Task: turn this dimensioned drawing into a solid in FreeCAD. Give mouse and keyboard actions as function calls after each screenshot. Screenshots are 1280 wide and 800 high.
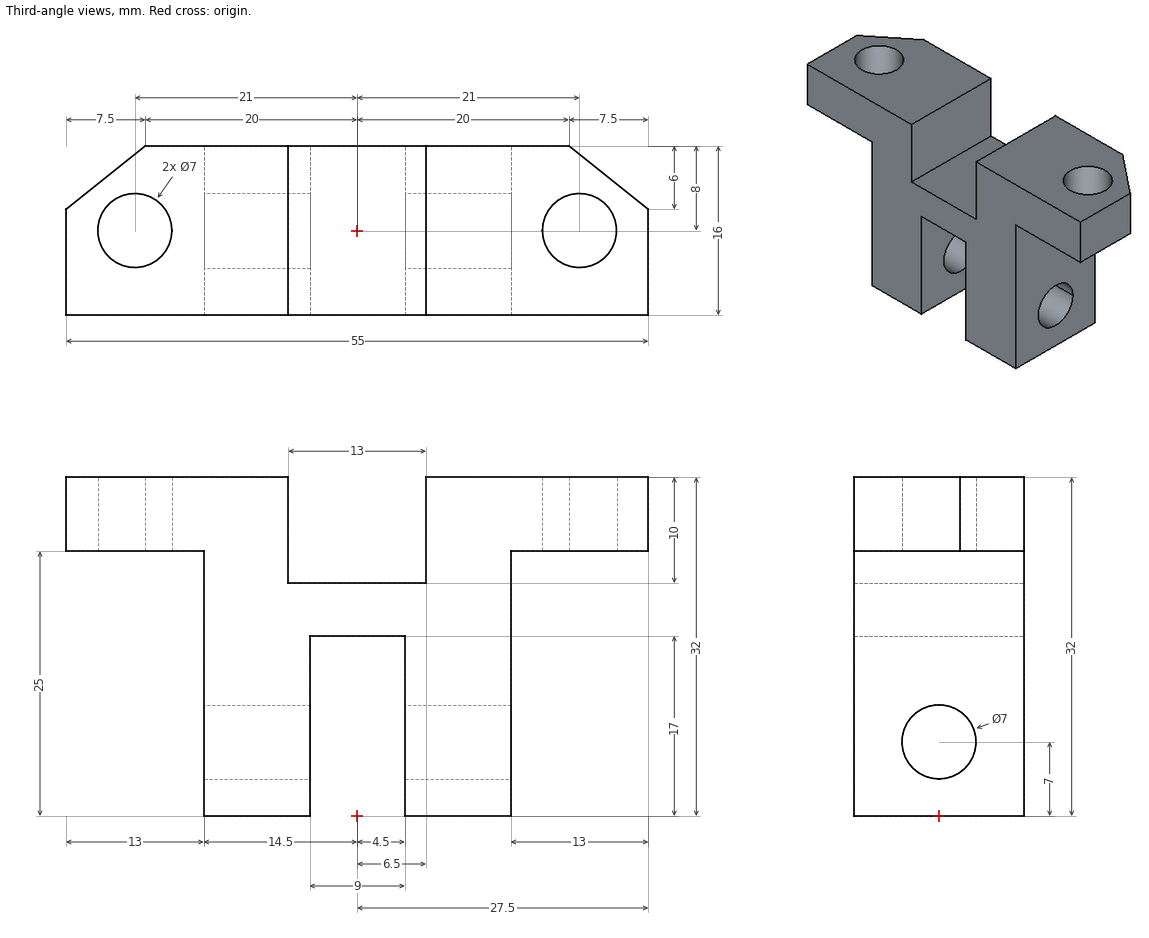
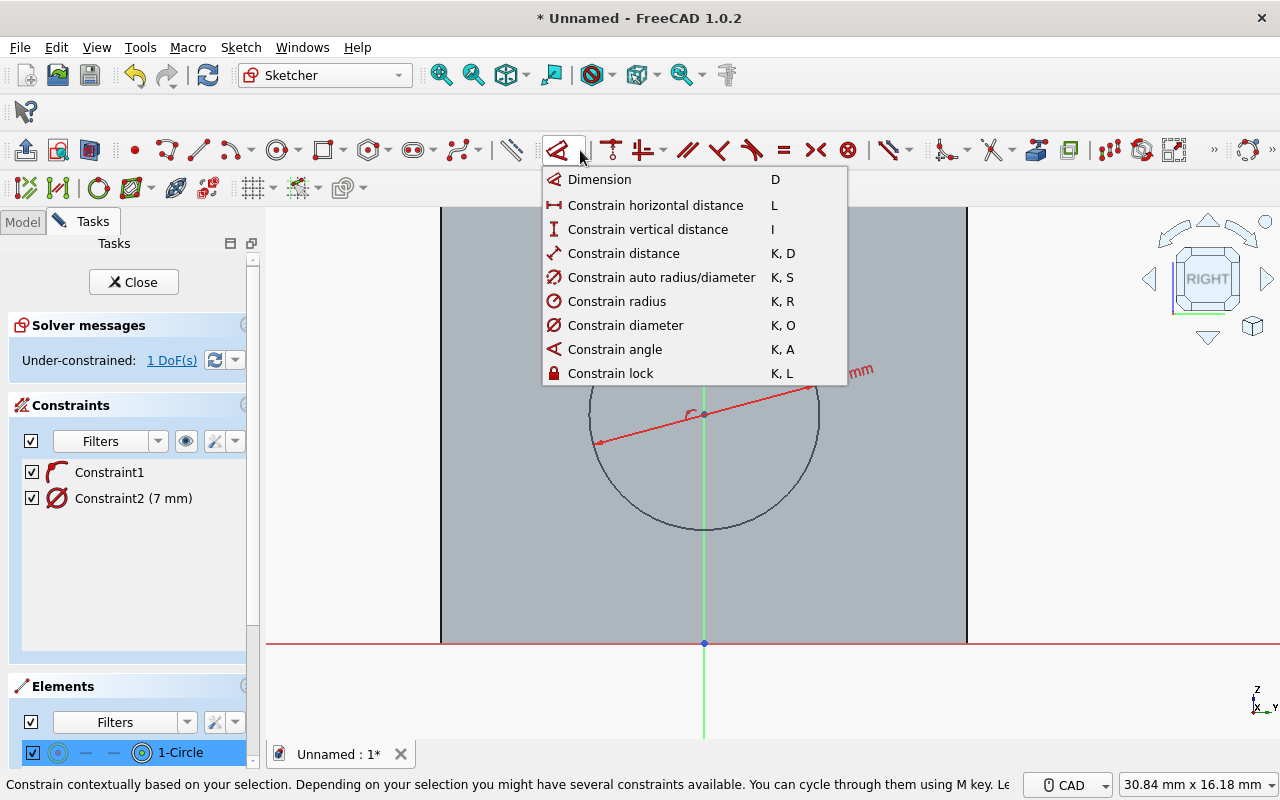
click(695, 229)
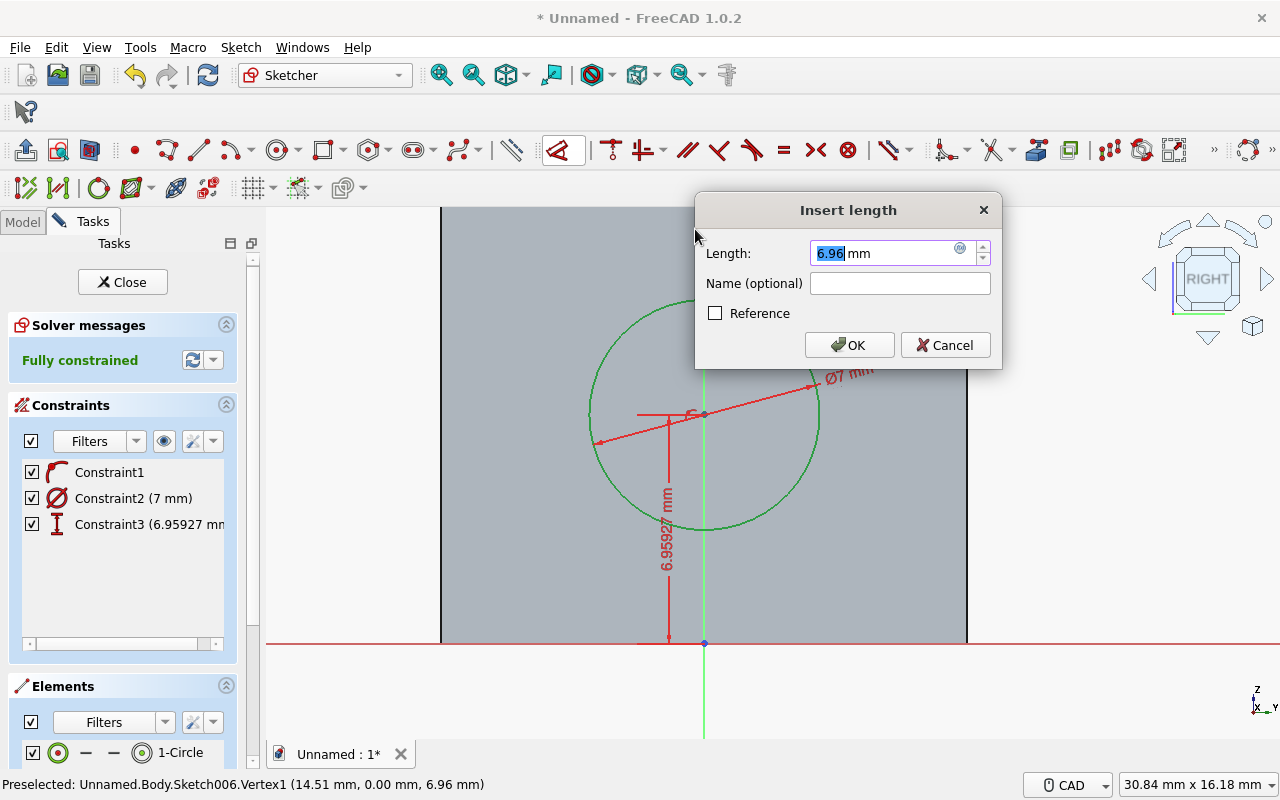
text(7)
key(Return)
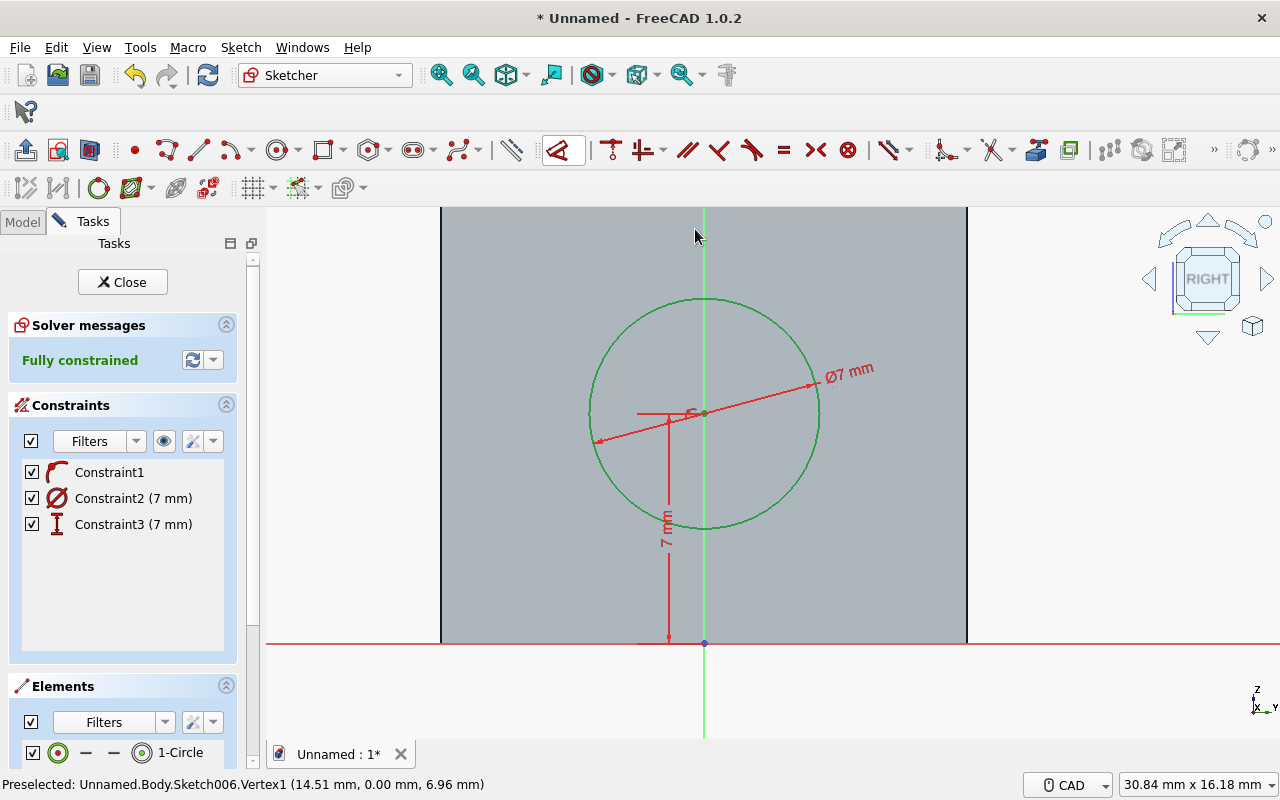
click(123, 282)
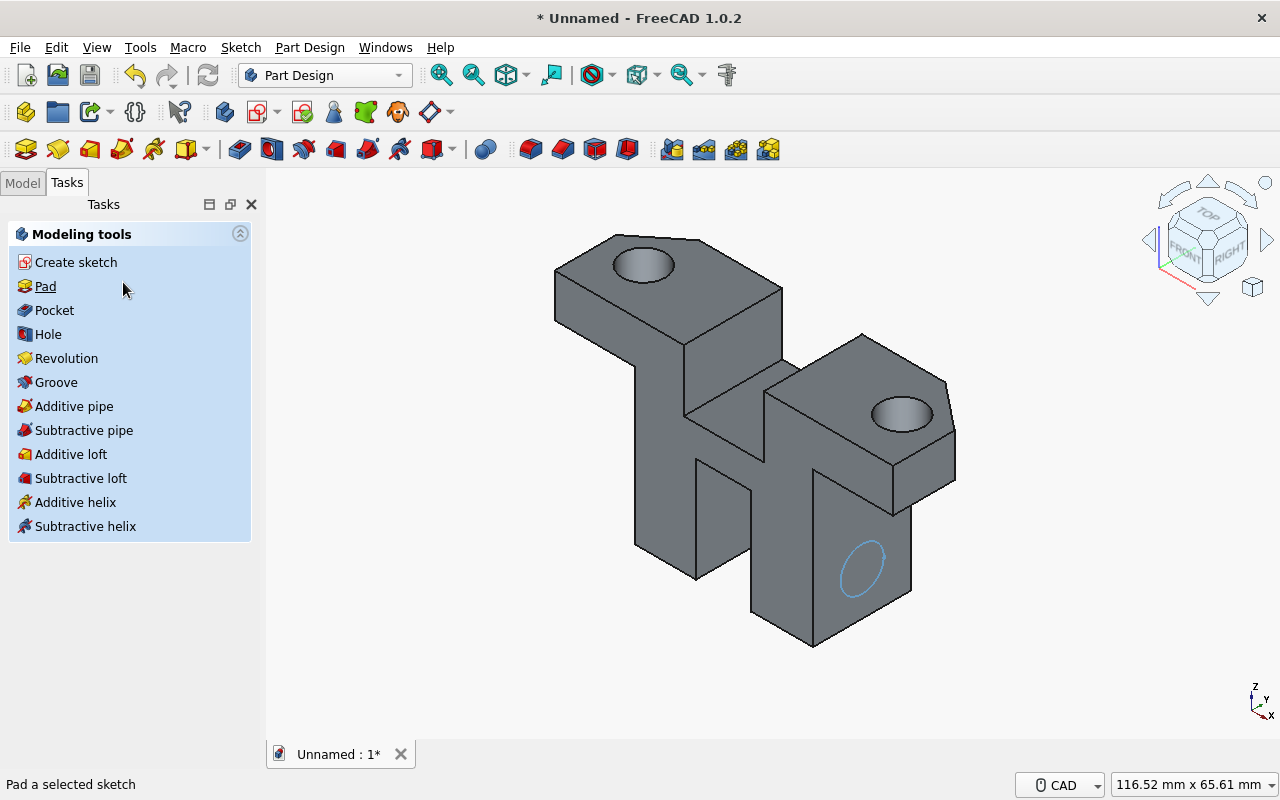
click(240, 150)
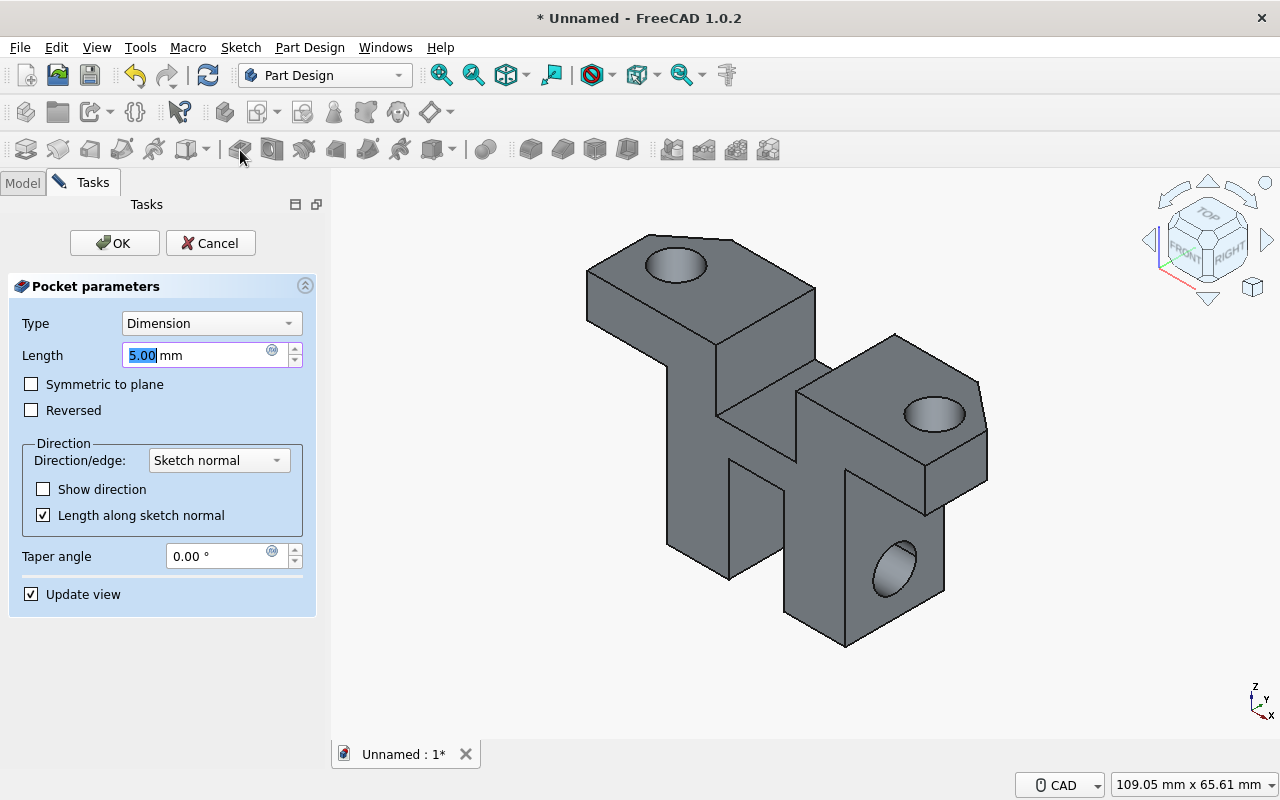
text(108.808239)
key(Tab)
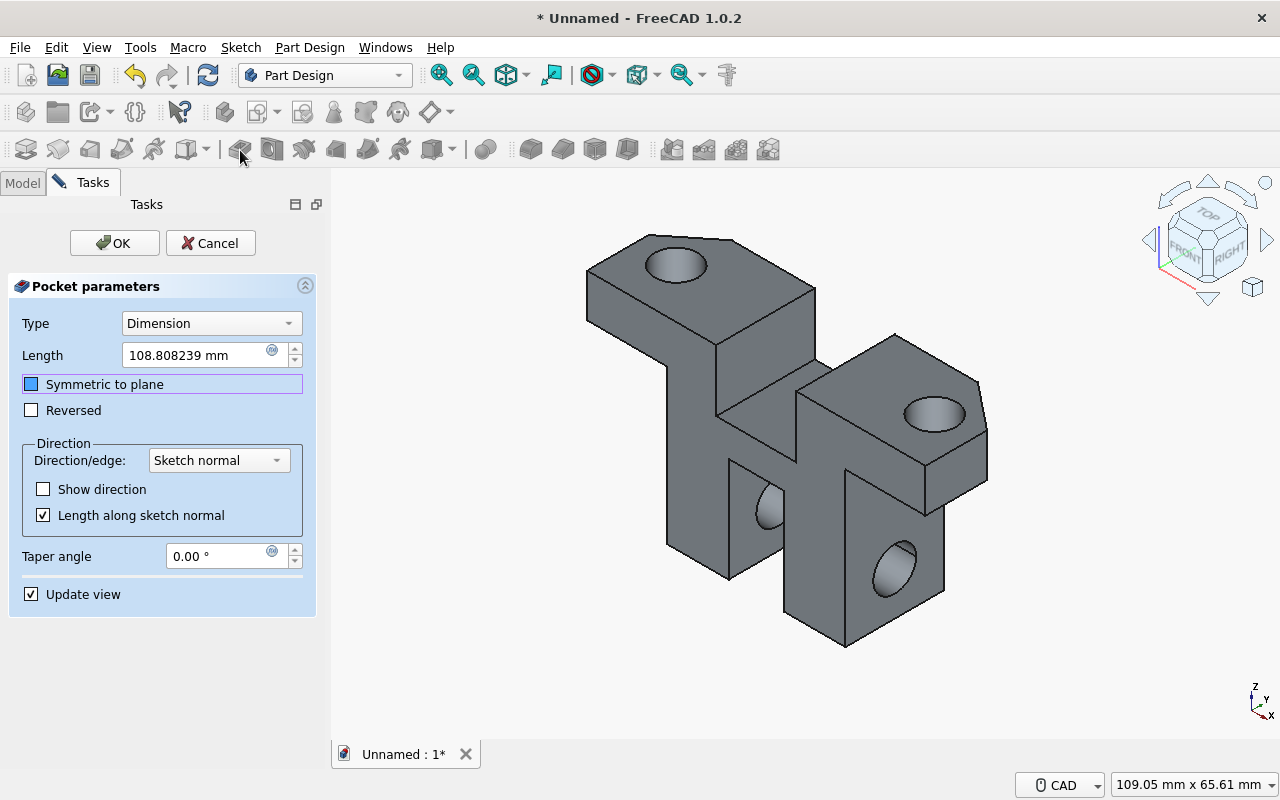
click(30, 384)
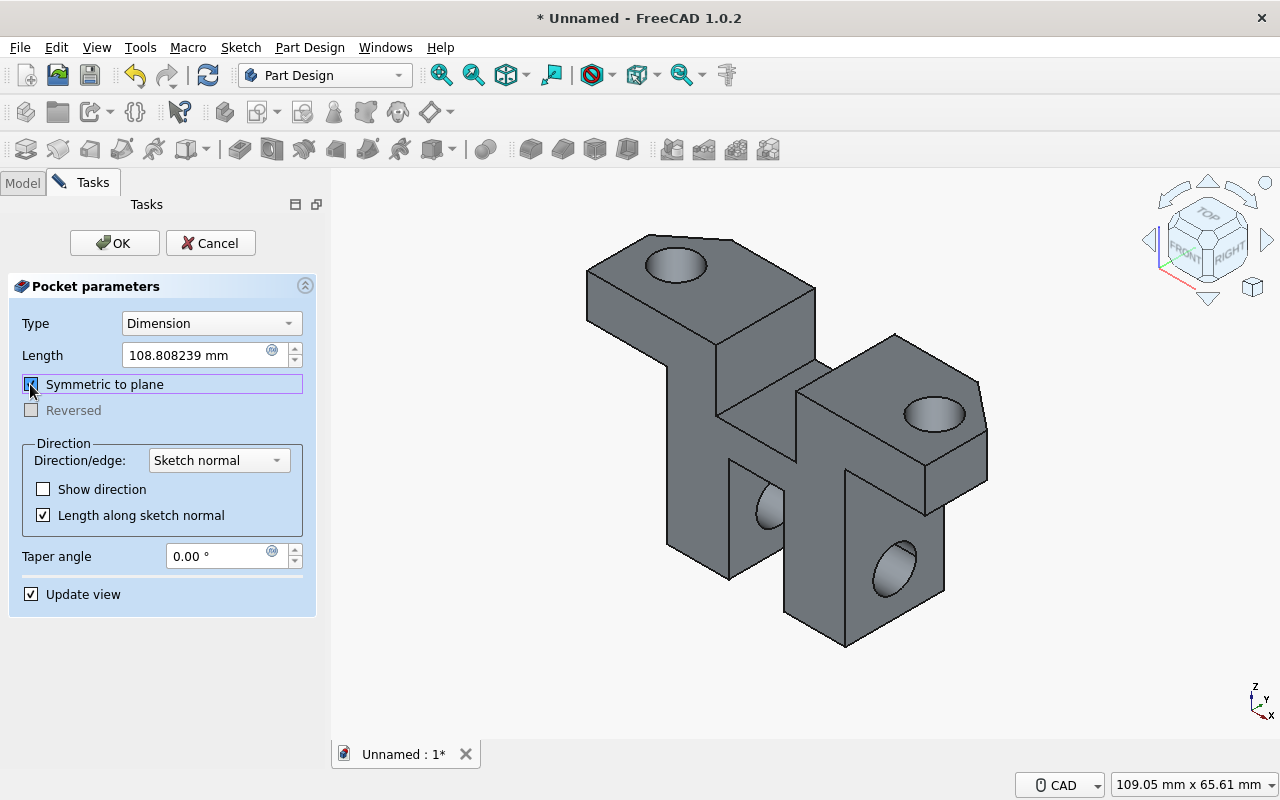
click(115, 243)